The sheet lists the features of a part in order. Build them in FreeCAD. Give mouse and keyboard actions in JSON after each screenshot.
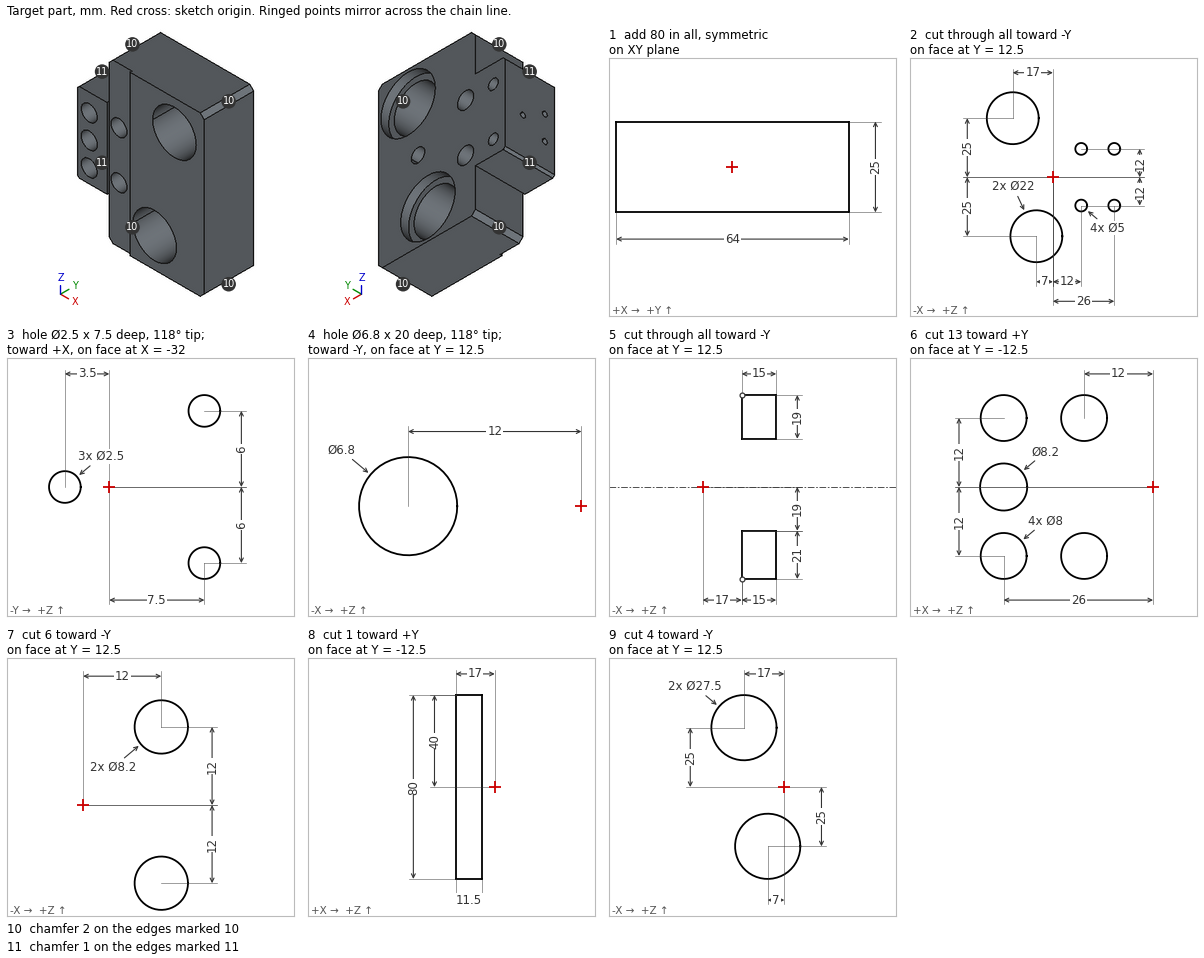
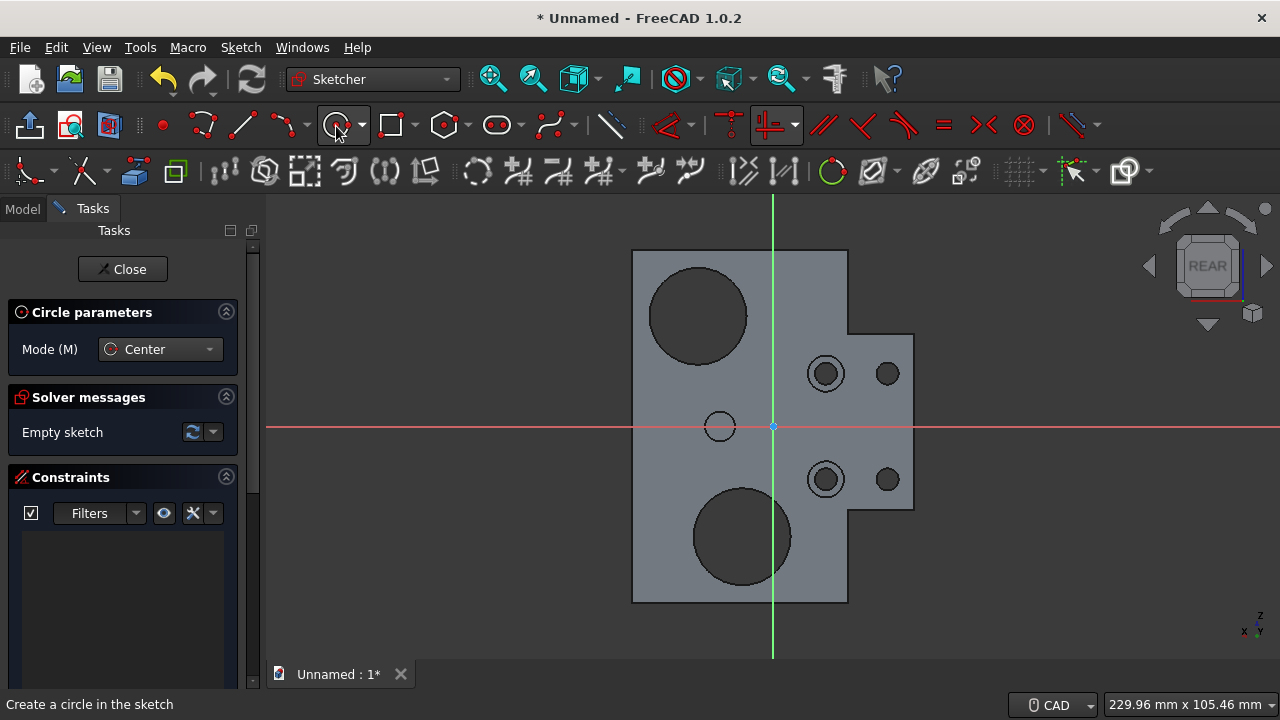
{"action": "left_click", "coordinate": [698, 316]}
{"action": "left_click", "coordinate": [741, 273]}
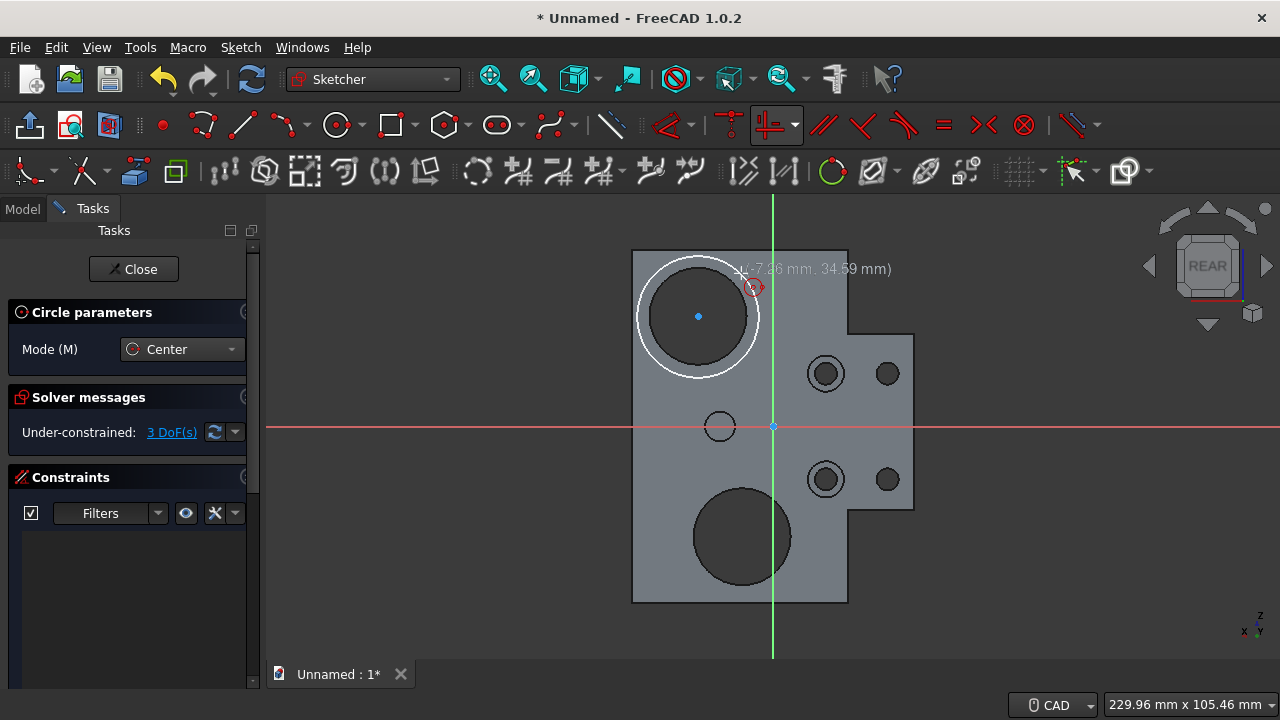
{"action": "left_click", "coordinate": [742, 537]}
{"action": "left_click", "coordinate": [699, 494]}
{"action": "key", "text": "Escape"}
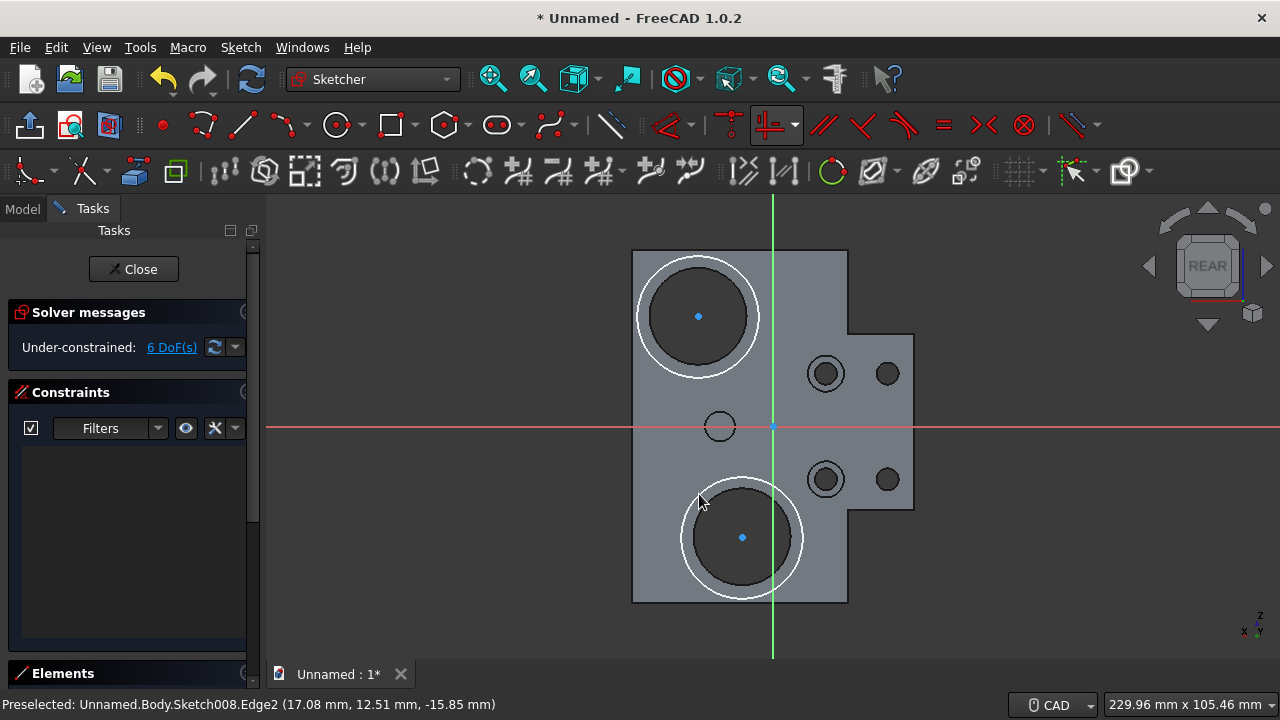
{"action": "left_click", "coordinate": [741, 274]}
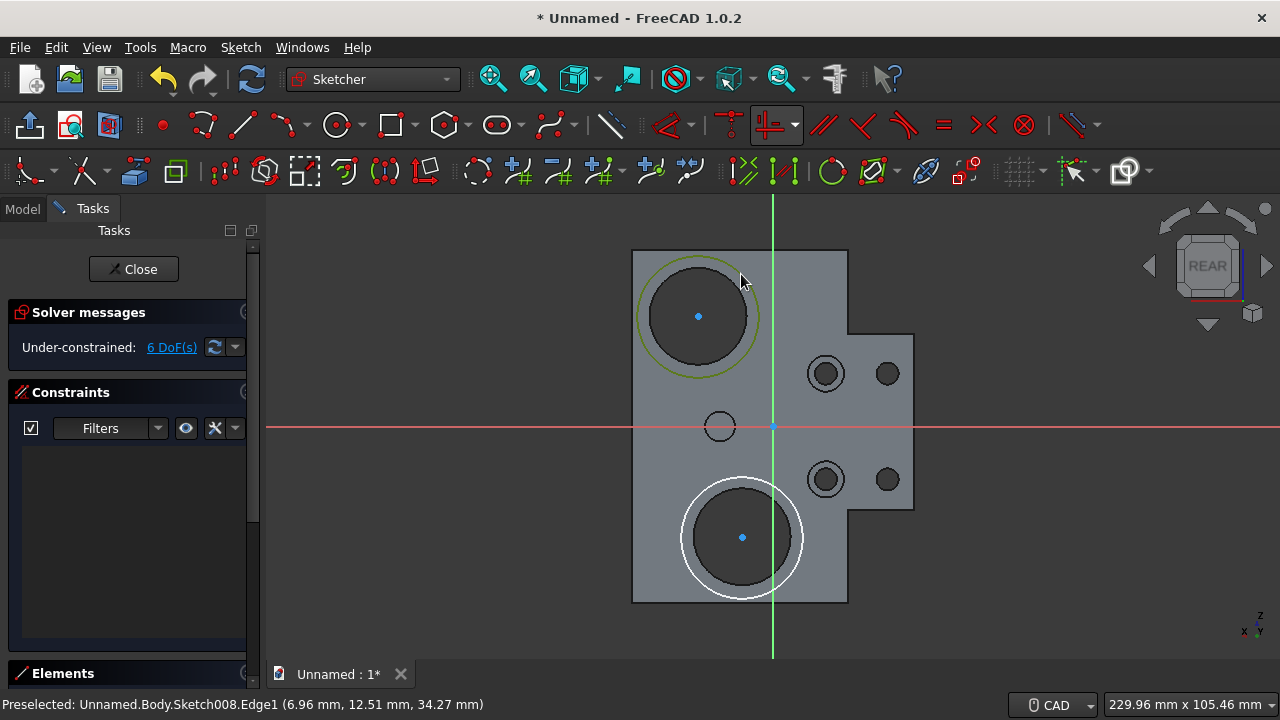
{"action": "left_click", "coordinate": [785, 495]}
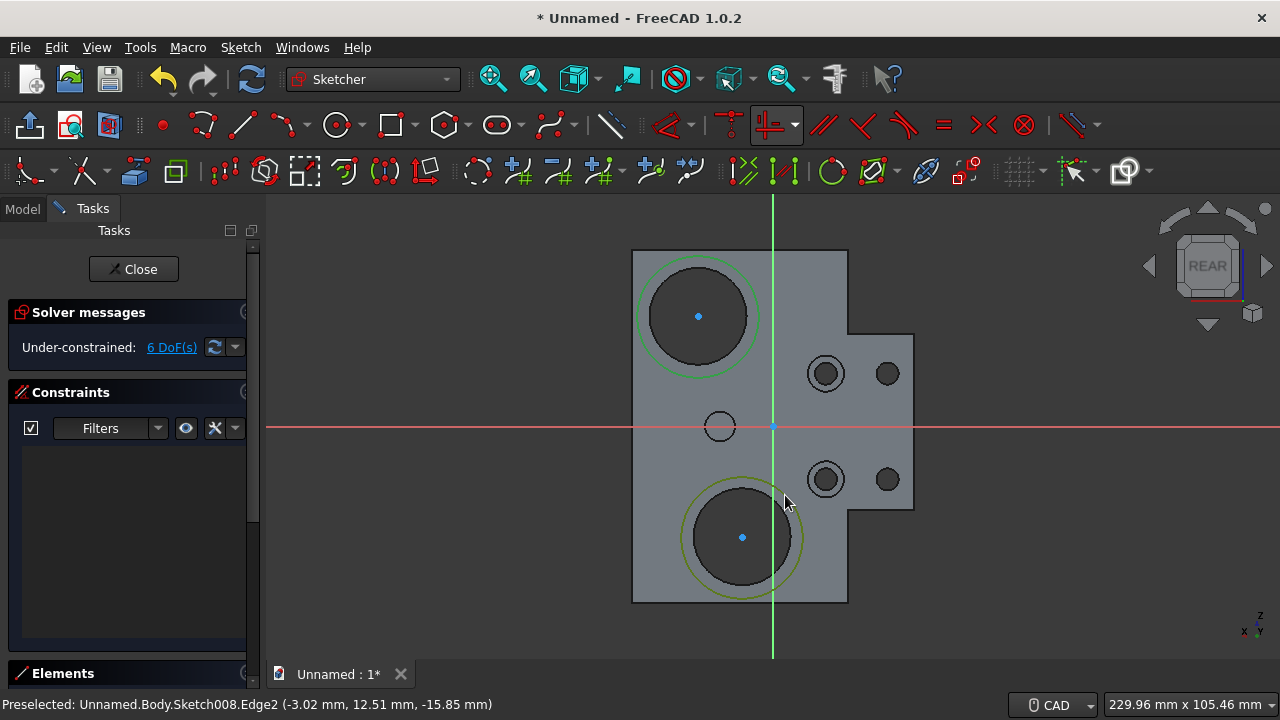
{"action": "left_click", "coordinate": [944, 126]}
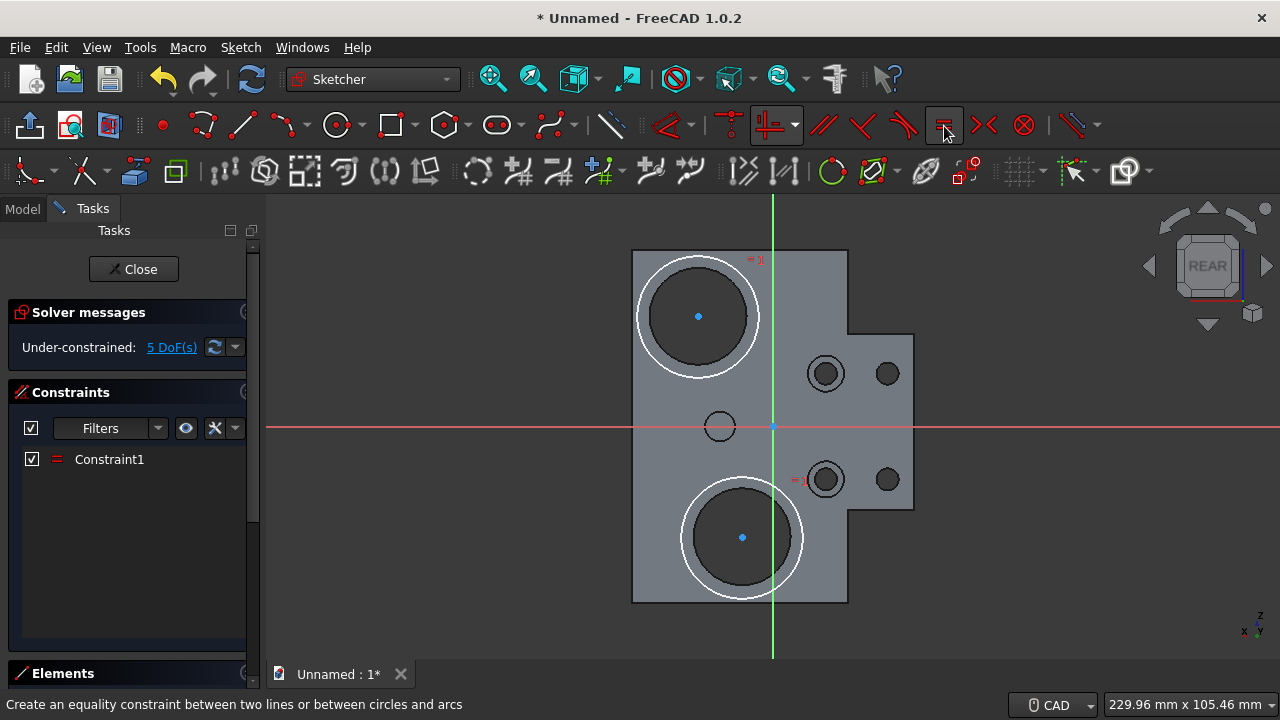
{"action": "left_click", "coordinate": [666, 126]}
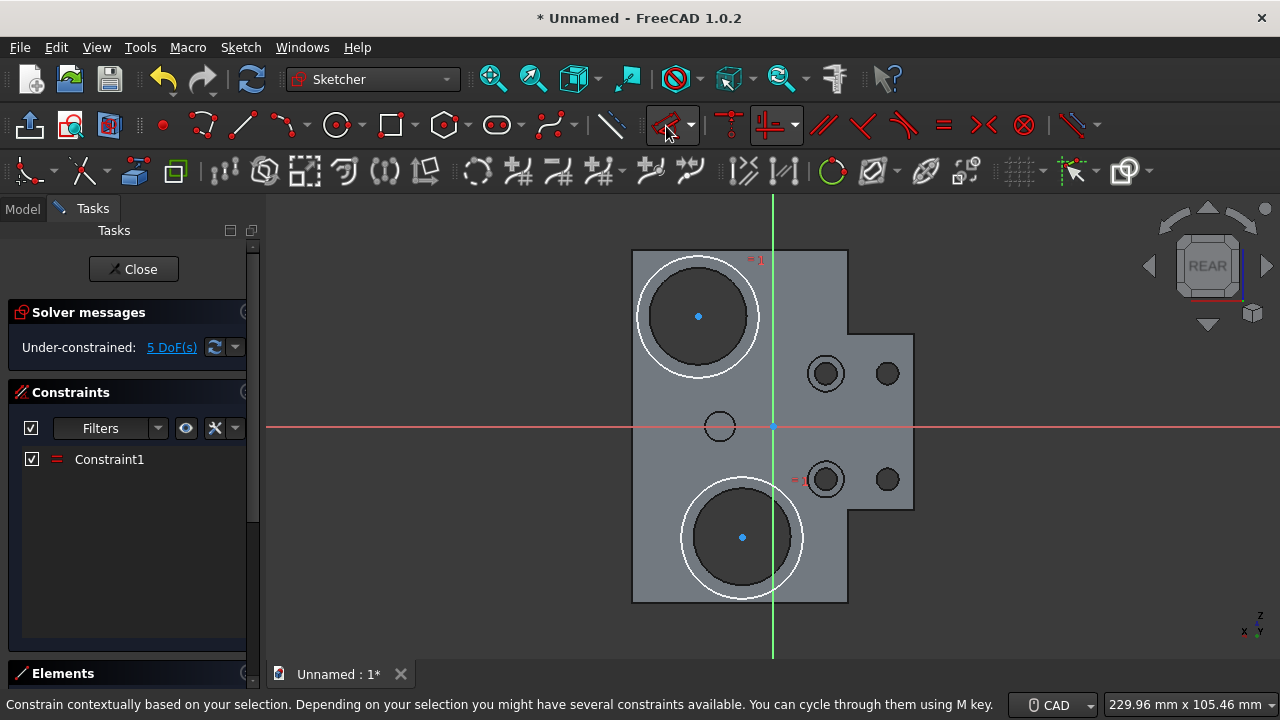
{"action": "left_click", "coordinate": [741, 274]}
{"action": "left_click", "coordinate": [787, 291]}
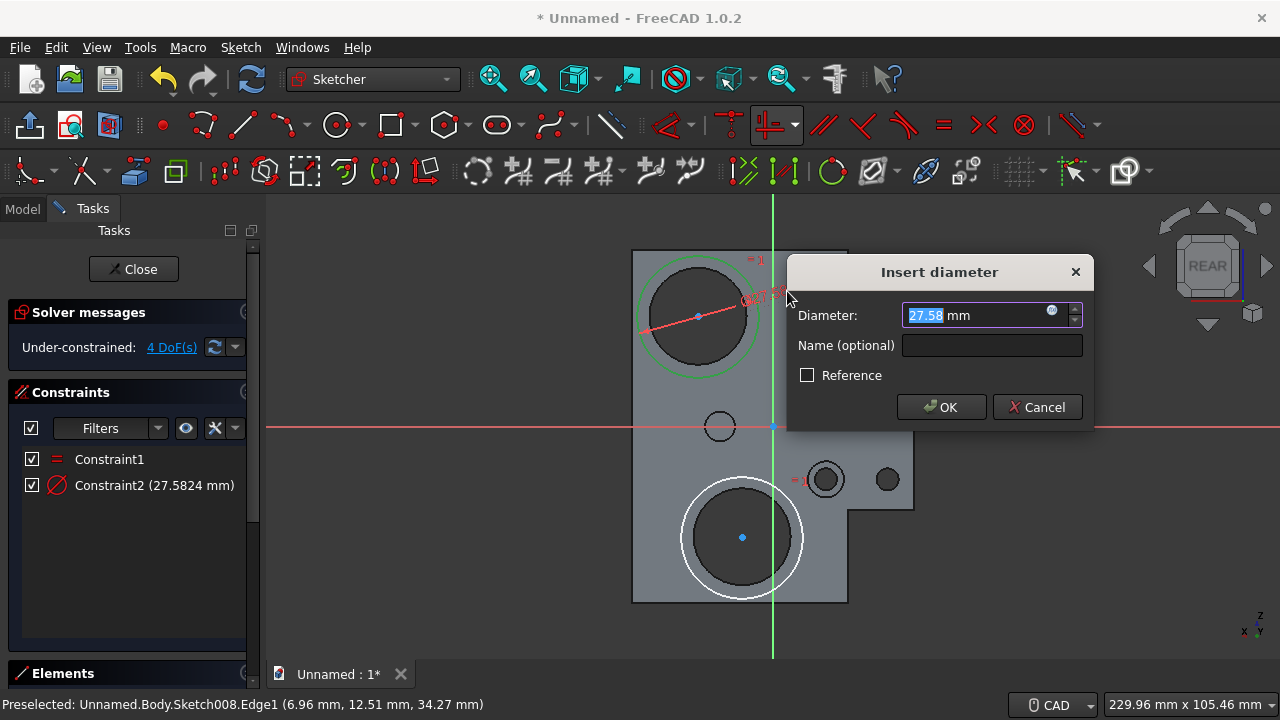
{"action": "type", "text": "27.5"}
{"action": "key", "text": "Return"}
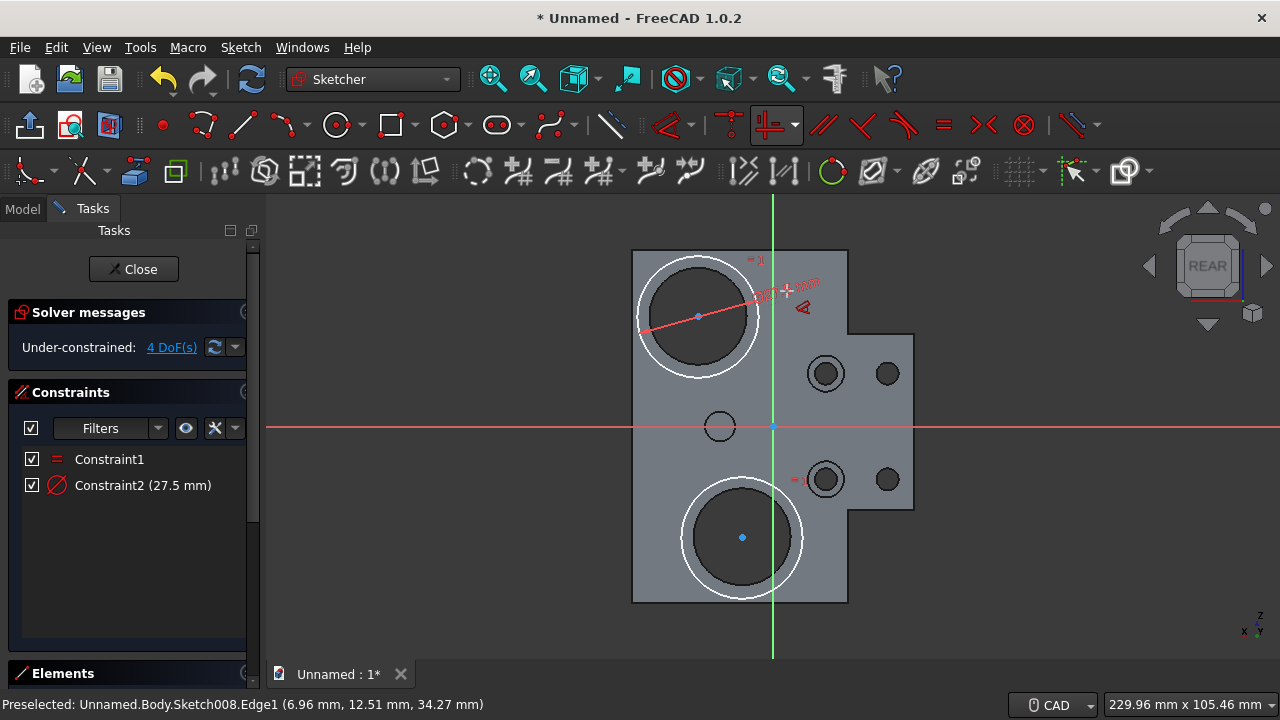
{"action": "scroll", "coordinate": [742, 538], "scroll_direction": "up", "scroll_amount": 2}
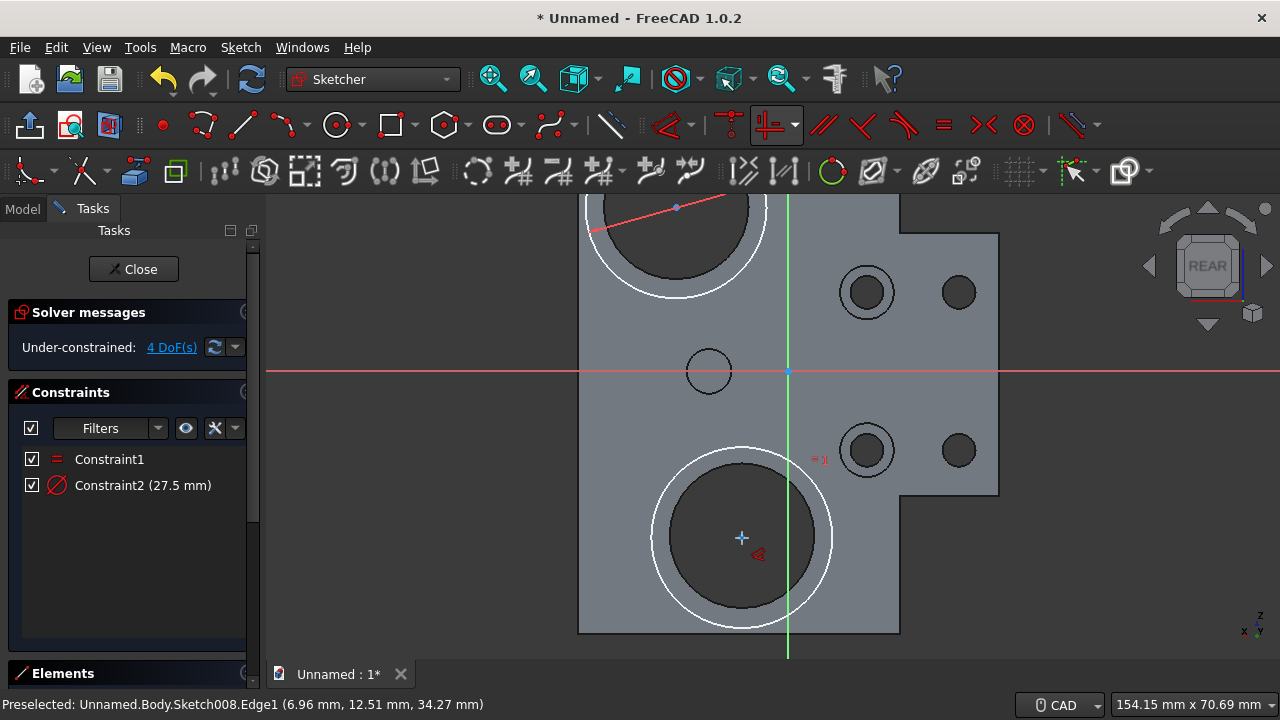
{"action": "left_click", "coordinate": [742, 538]}
{"action": "left_click", "coordinate": [765, 572]}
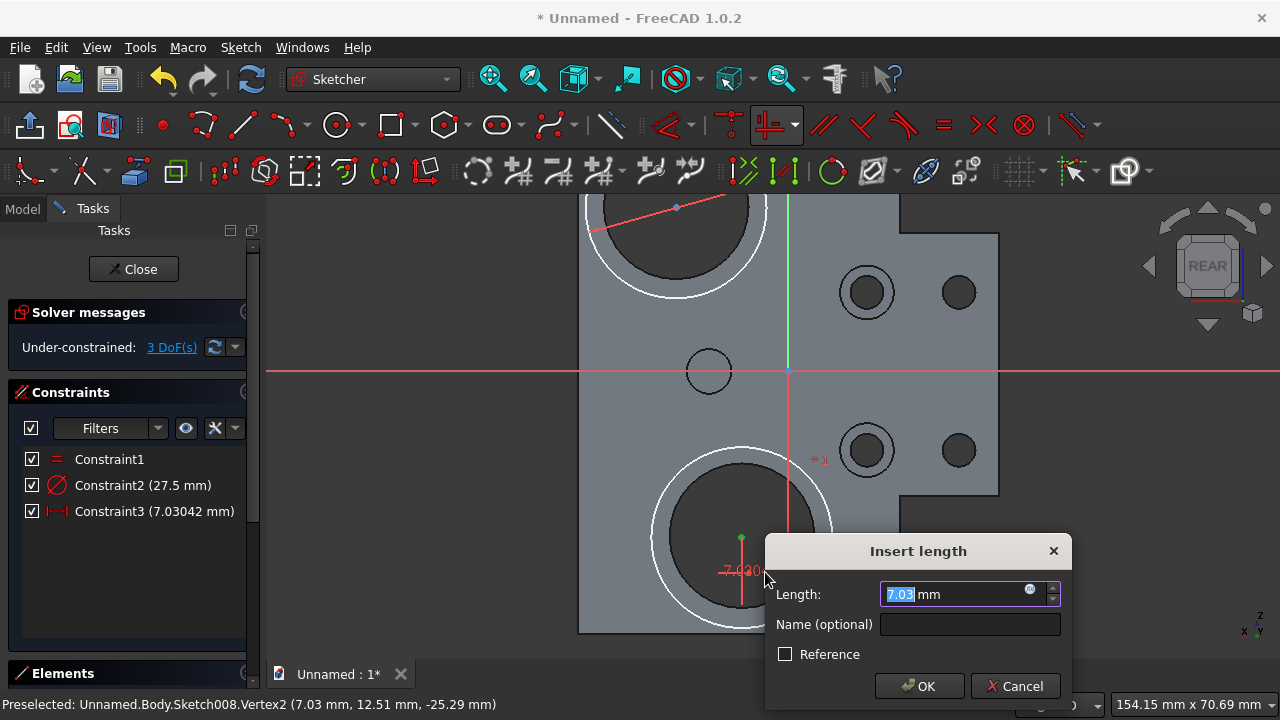
{"action": "type", "text": "7"}
{"action": "key", "text": "Return"}